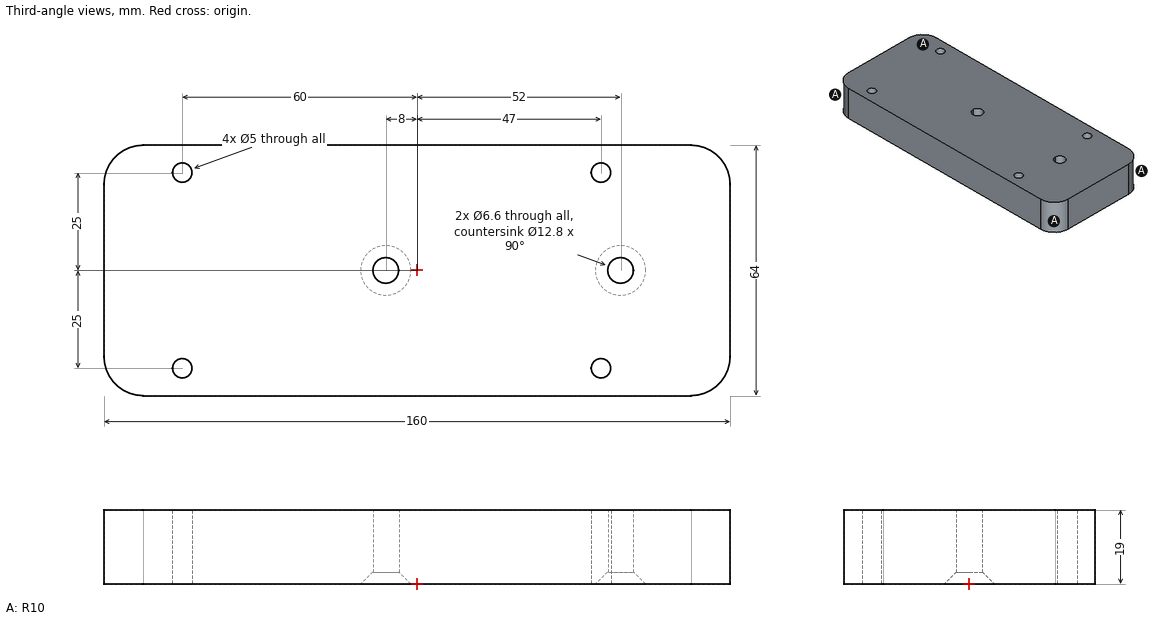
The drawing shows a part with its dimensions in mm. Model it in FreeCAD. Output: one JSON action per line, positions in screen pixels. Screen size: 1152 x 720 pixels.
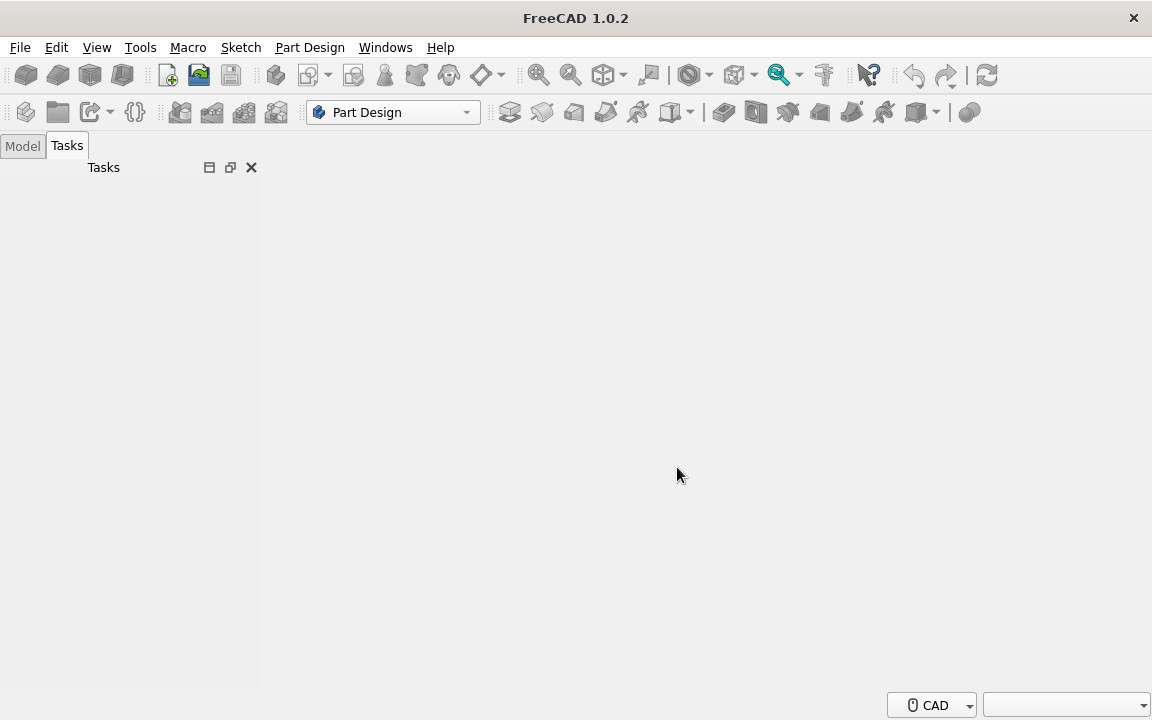
{"action": "left_click", "coordinate": [168, 76]}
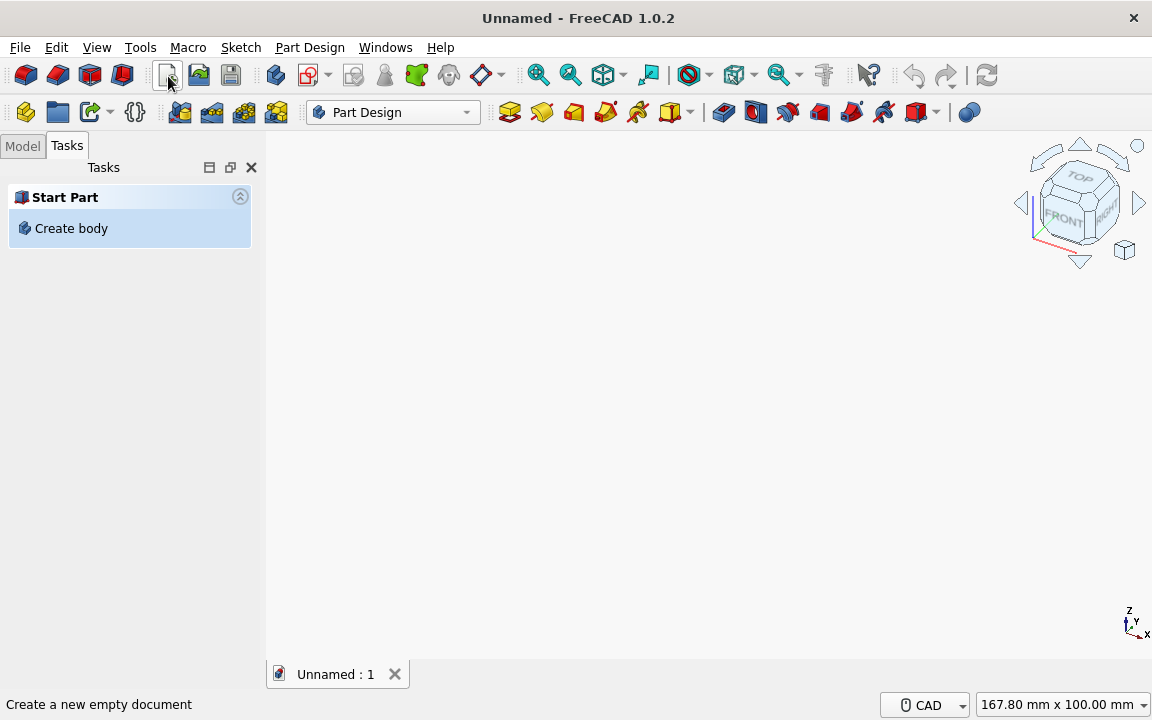
{"action": "left_click", "coordinate": [308, 76]}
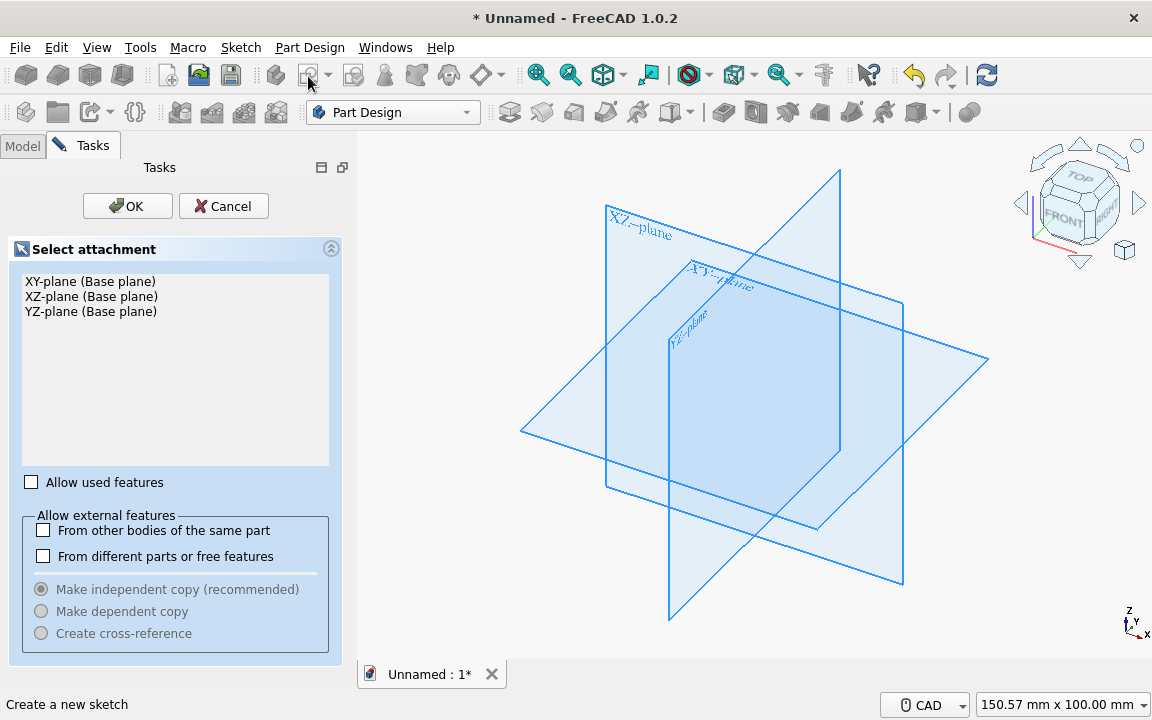
{"action": "left_click", "coordinate": [82, 282]}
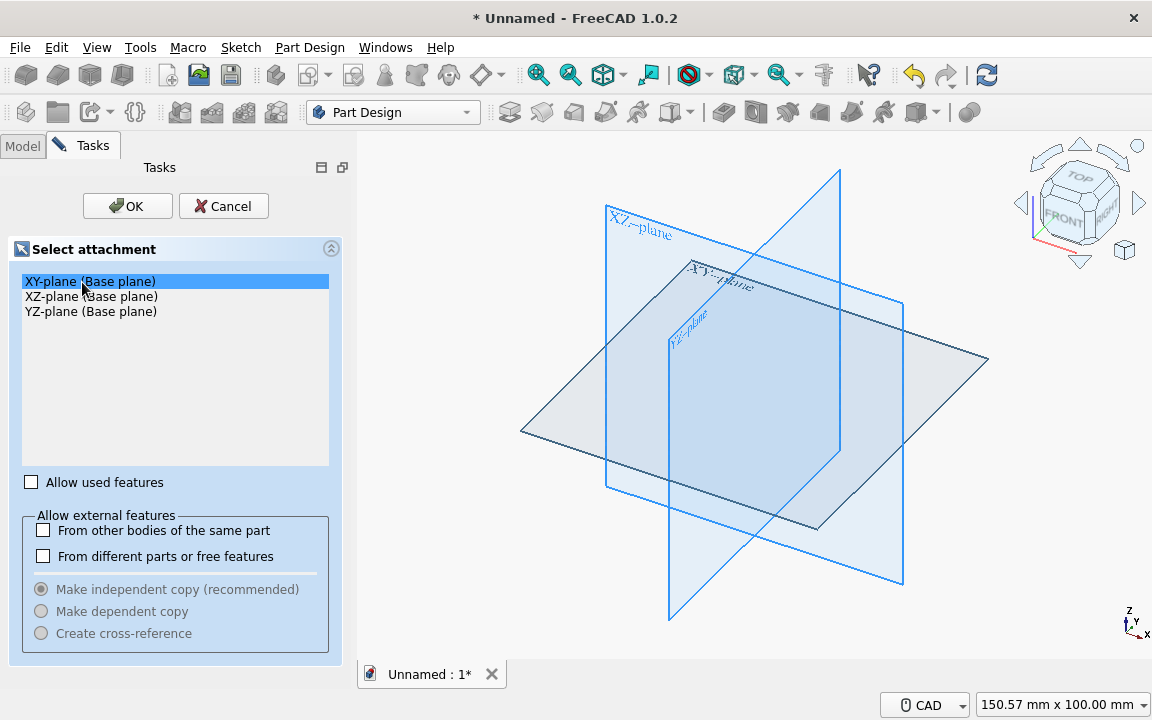
{"action": "left_click", "coordinate": [128, 206]}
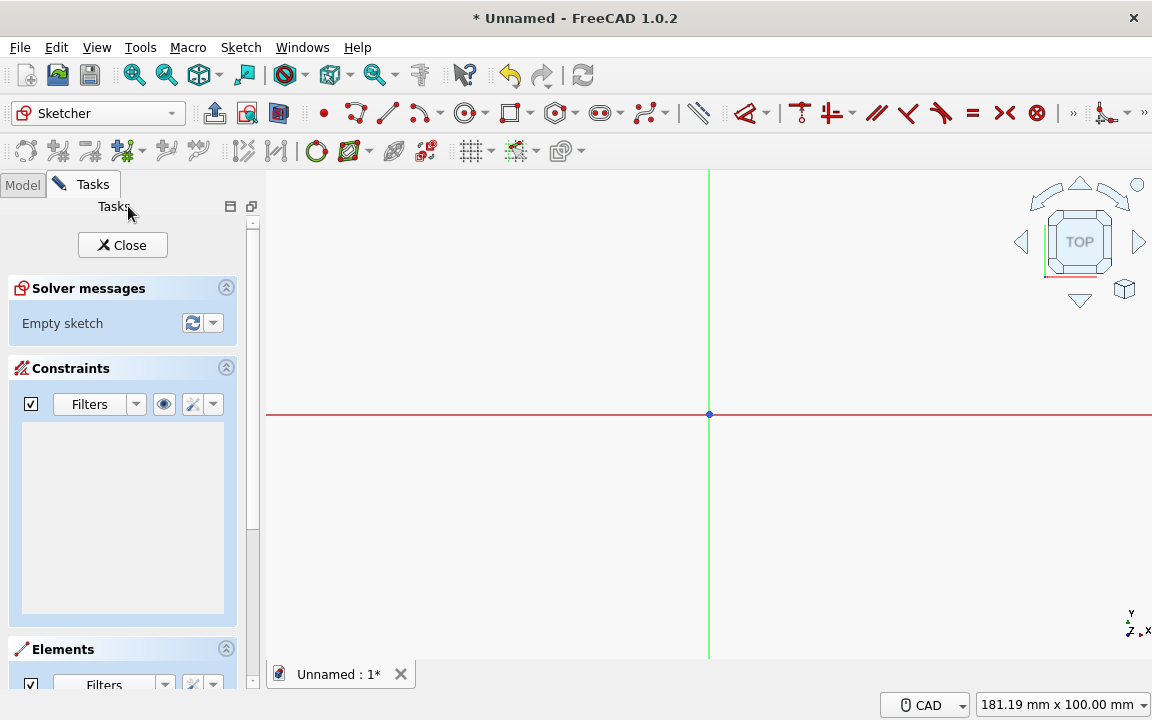
{"action": "scroll", "coordinate": [501, 414], "scroll_direction": "down", "scroll_amount": 2}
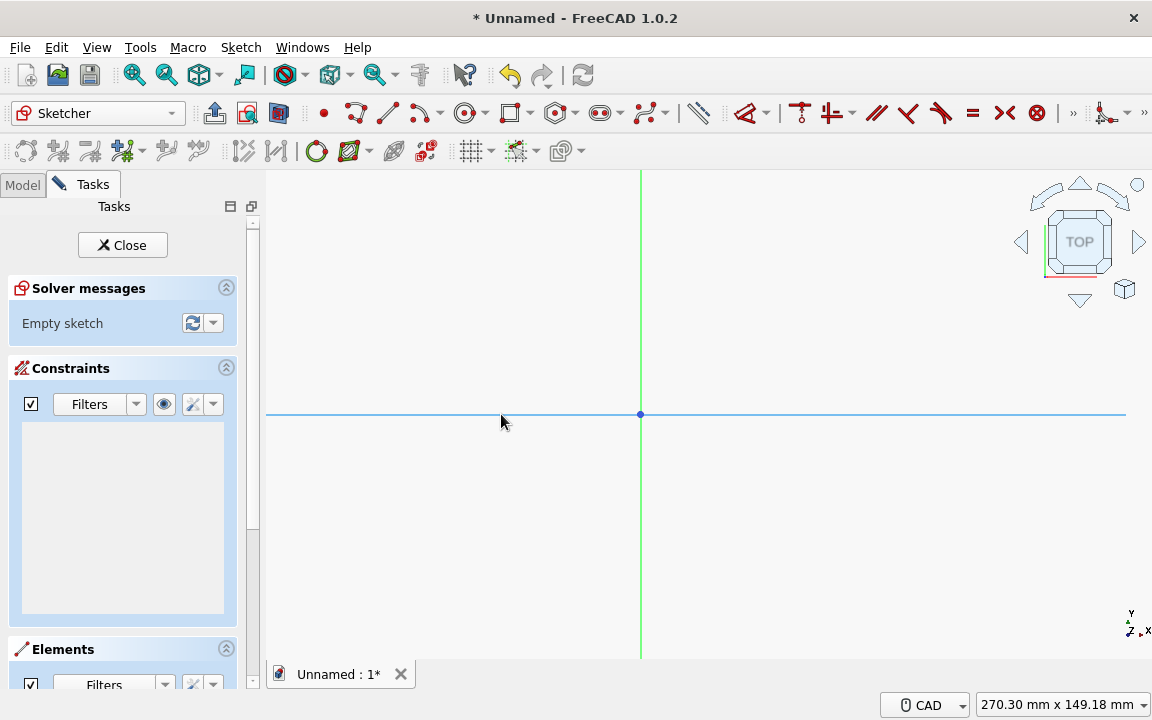
{"action": "left_click", "coordinate": [532, 114]}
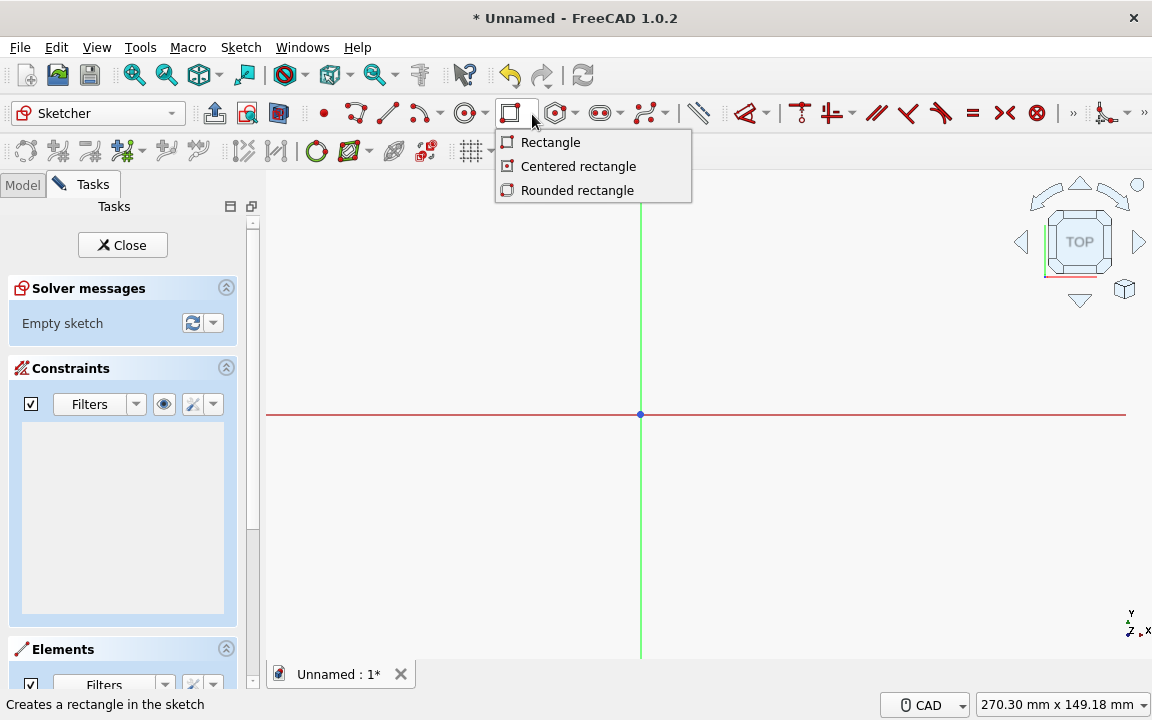
{"action": "left_click", "coordinate": [594, 166]}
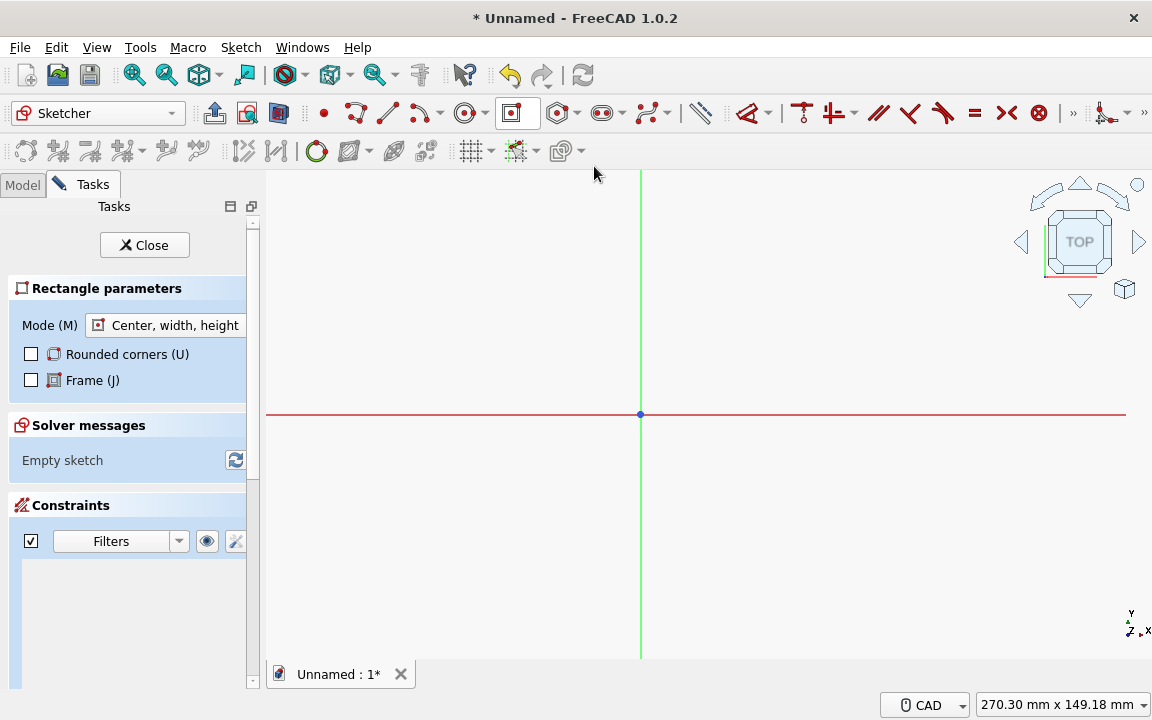
{"action": "left_click", "coordinate": [641, 414]}
{"action": "left_click", "coordinate": [903, 310]}
{"action": "key", "text": "Escape"}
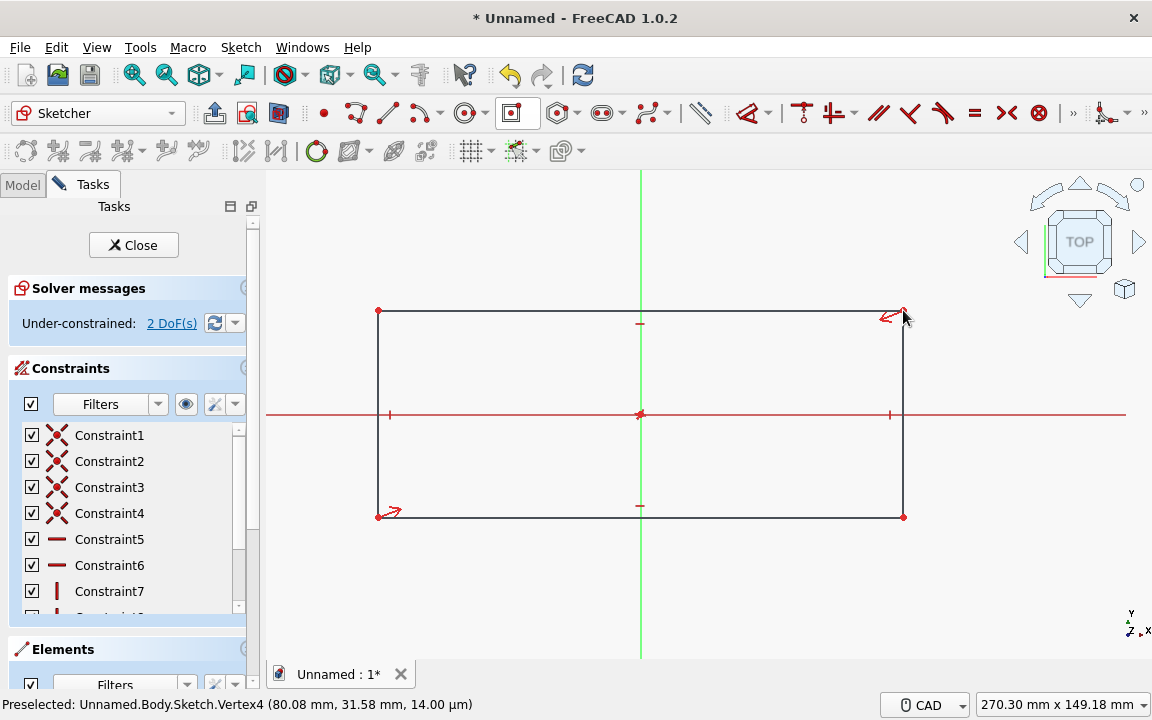
{"action": "left_click", "coordinate": [748, 114]}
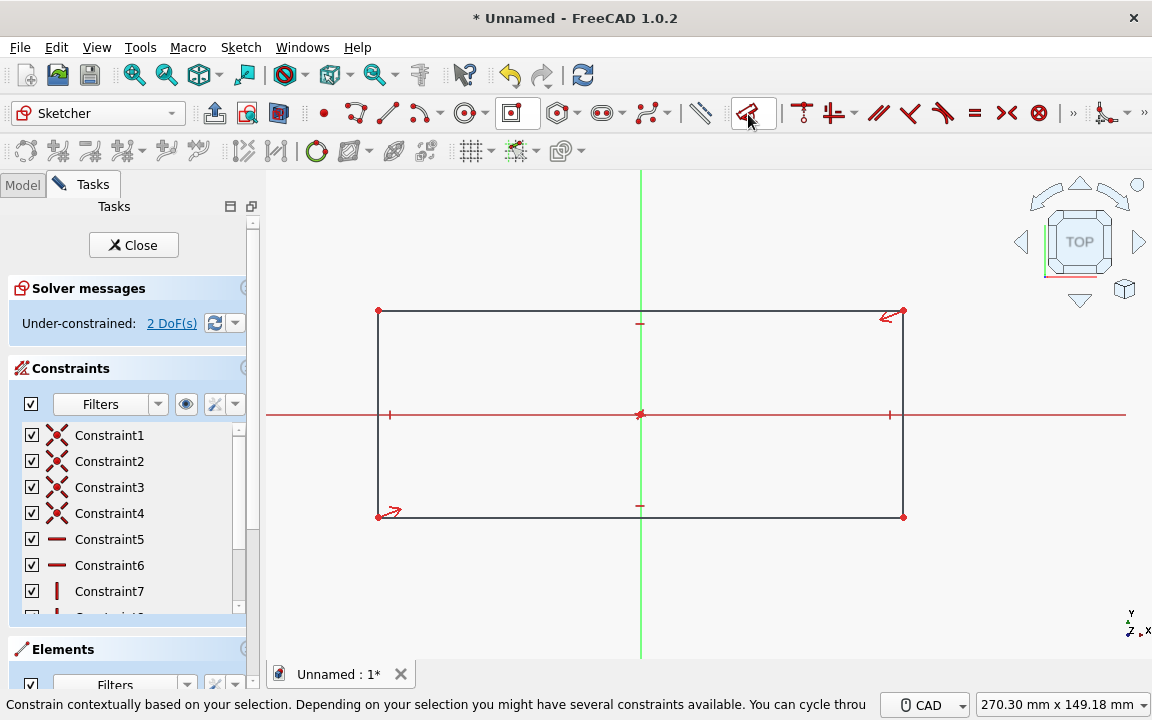
{"action": "left_click", "coordinate": [903, 456]}
{"action": "left_click", "coordinate": [937, 367]}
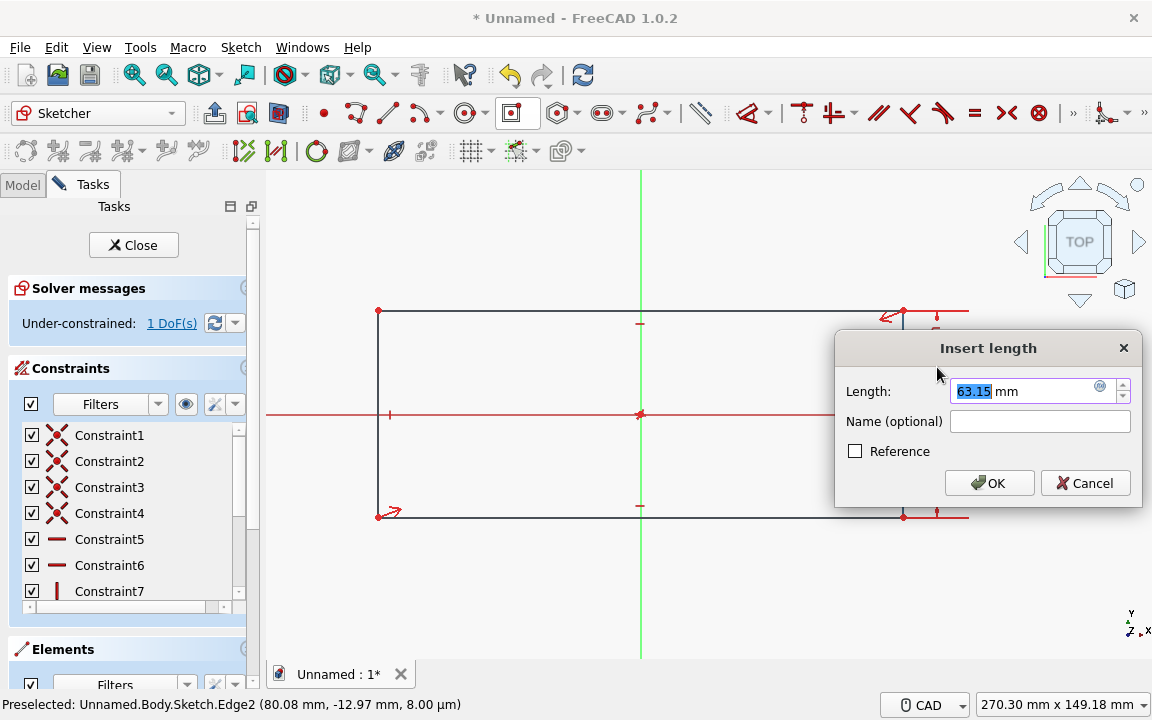
{"action": "type", "text": "64"}
{"action": "key", "text": "Return"}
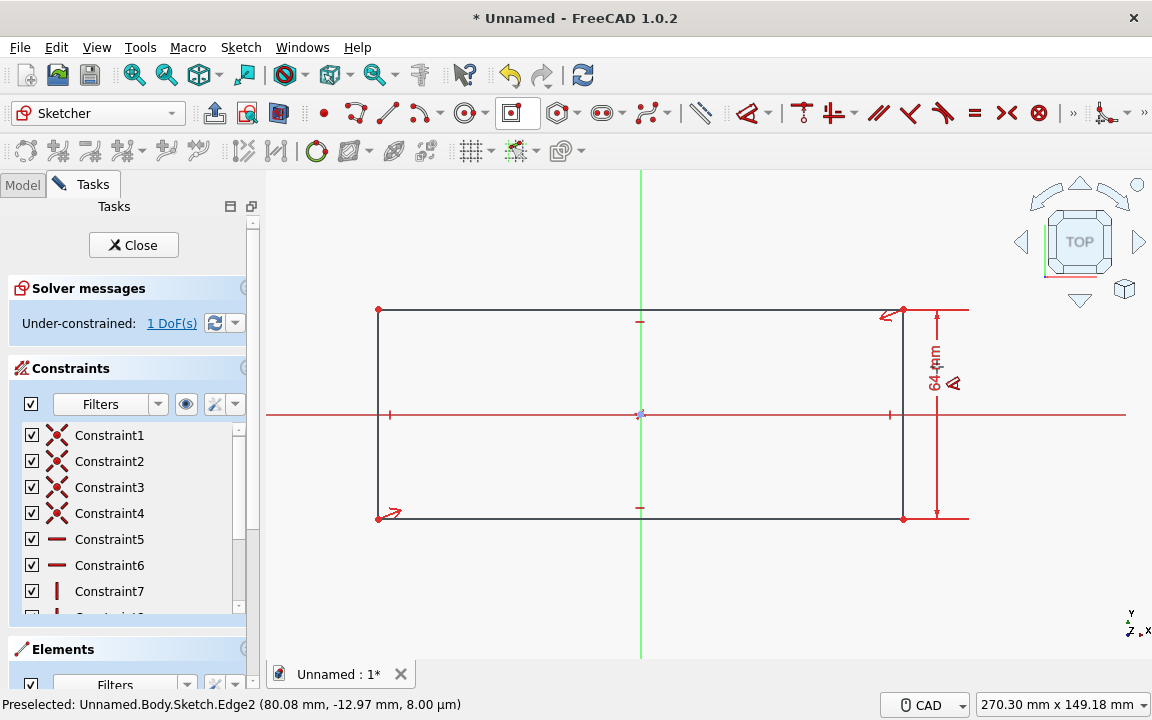
{"action": "left_click", "coordinate": [536, 519]}
{"action": "left_click", "coordinate": [520, 553]}